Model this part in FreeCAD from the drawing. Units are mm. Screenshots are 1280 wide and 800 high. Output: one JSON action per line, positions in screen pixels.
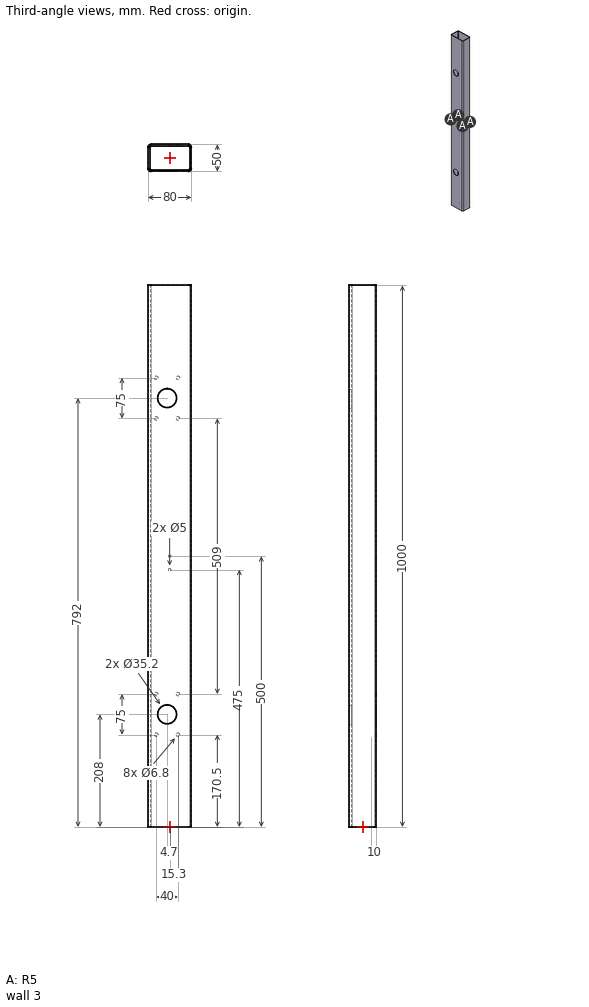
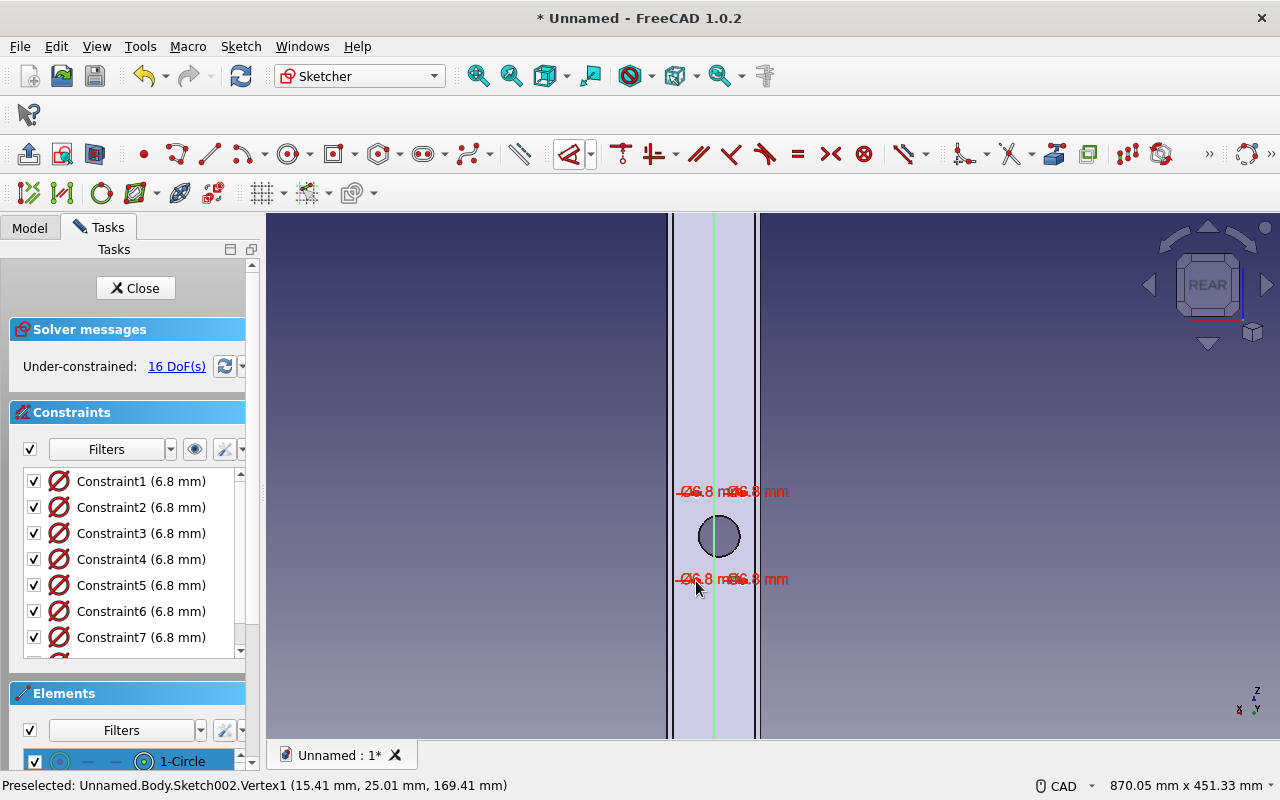
{"action": "left_click", "coordinate": [743, 581]}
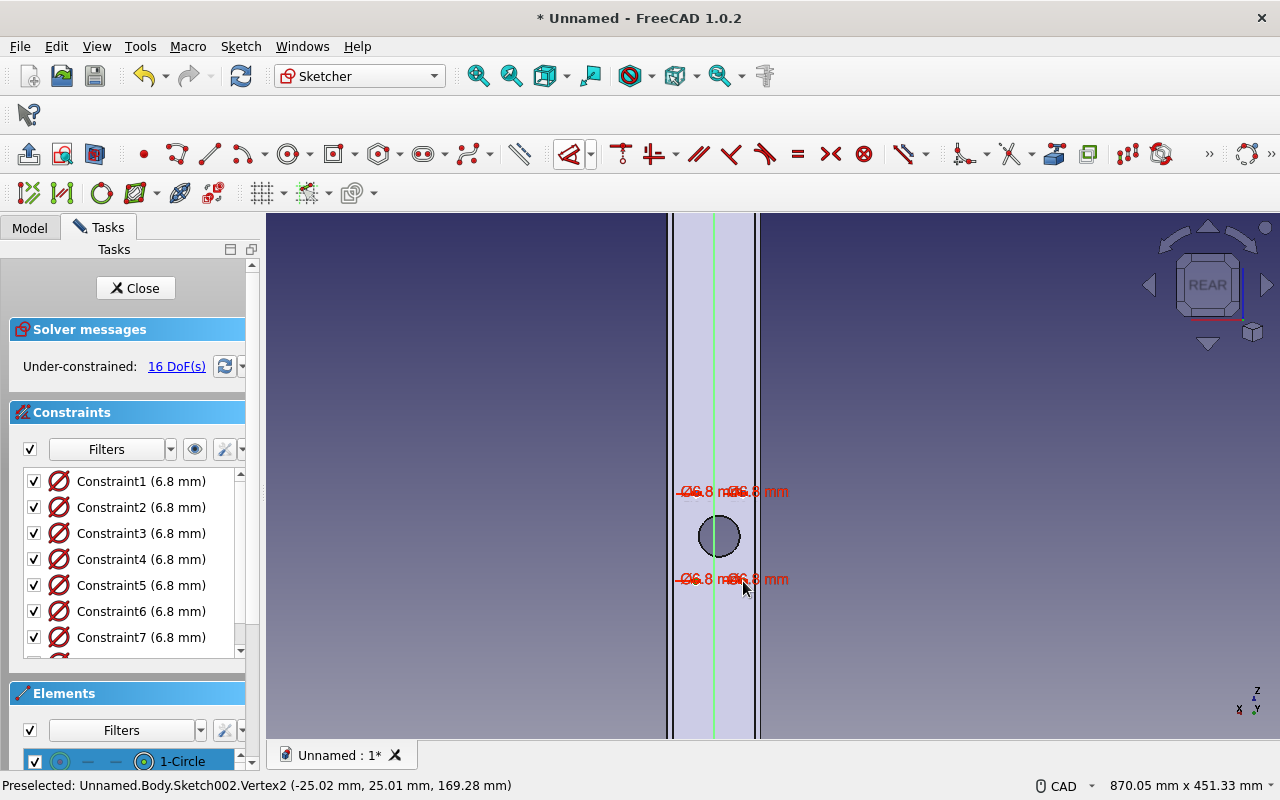
{"action": "left_click", "coordinate": [590, 154]}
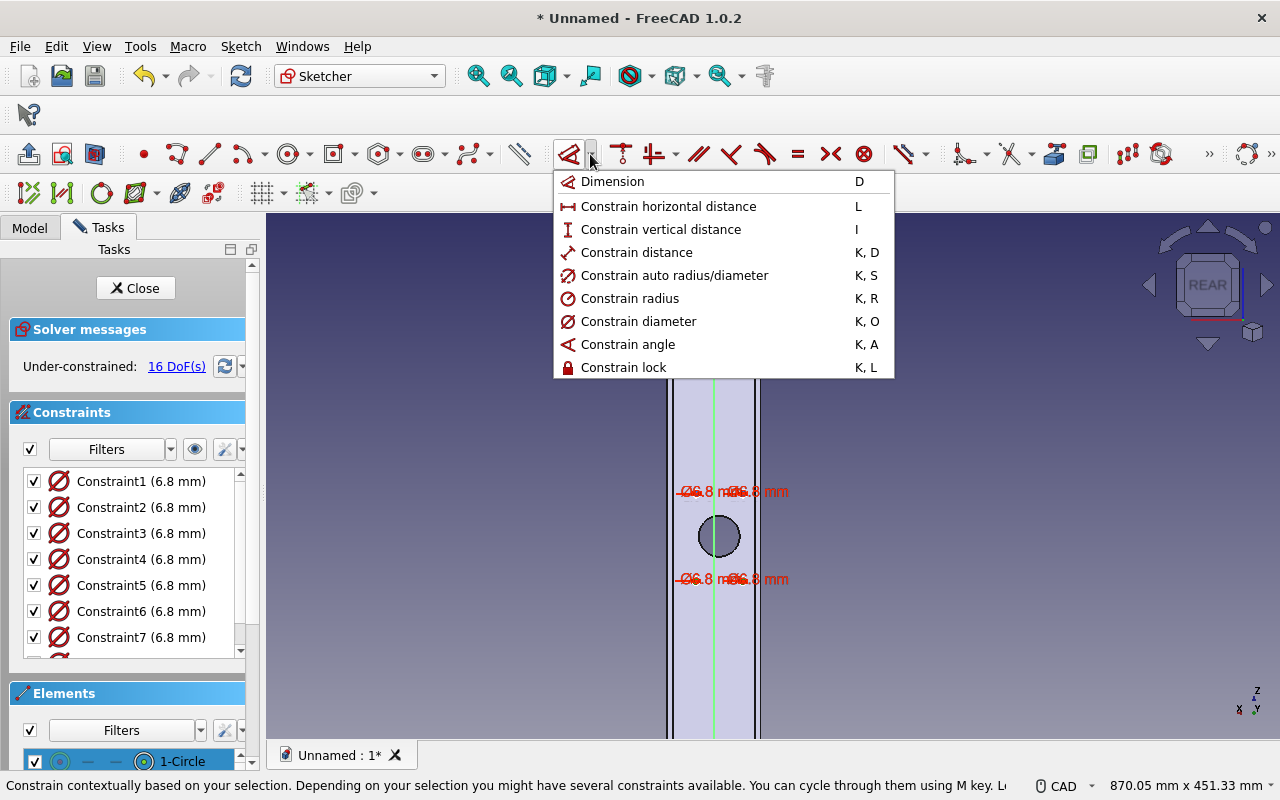
{"action": "left_click", "coordinate": [724, 206]}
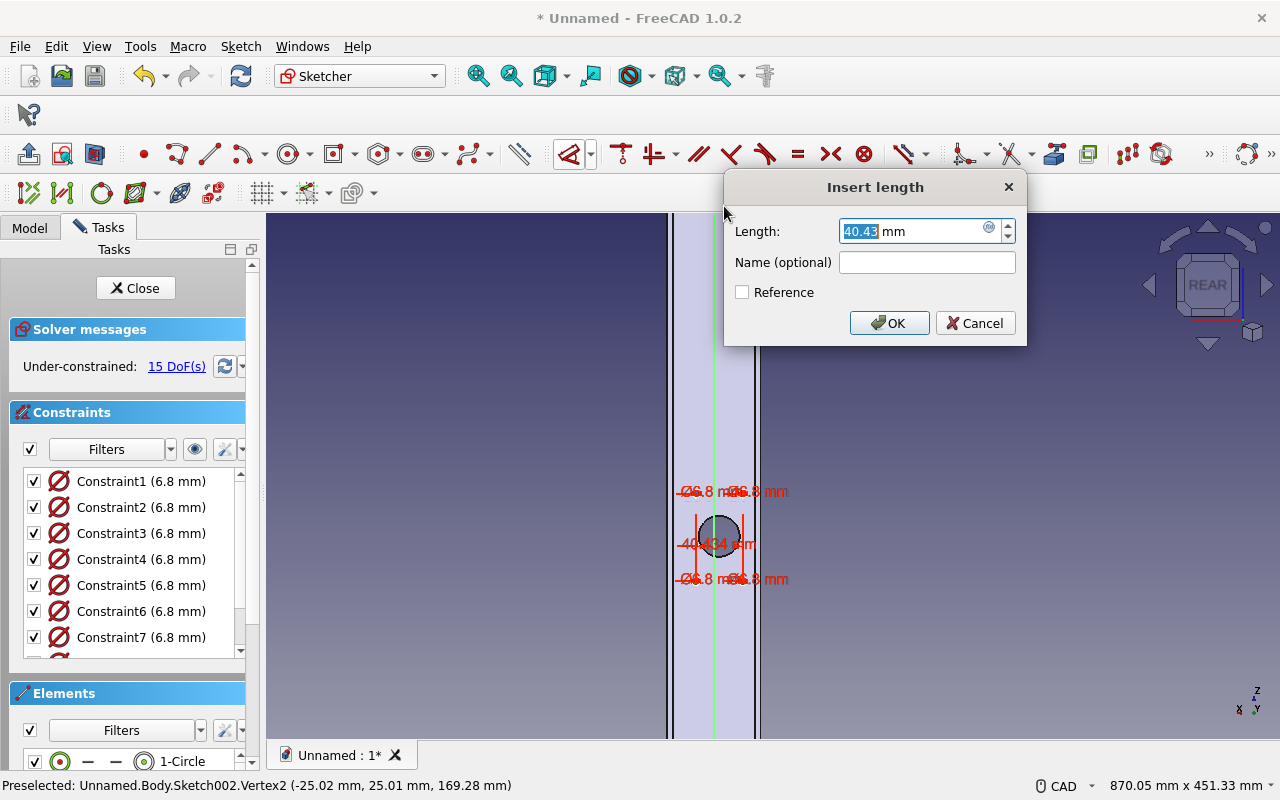
{"action": "type", "text": "40"}
{"action": "key", "text": "Return"}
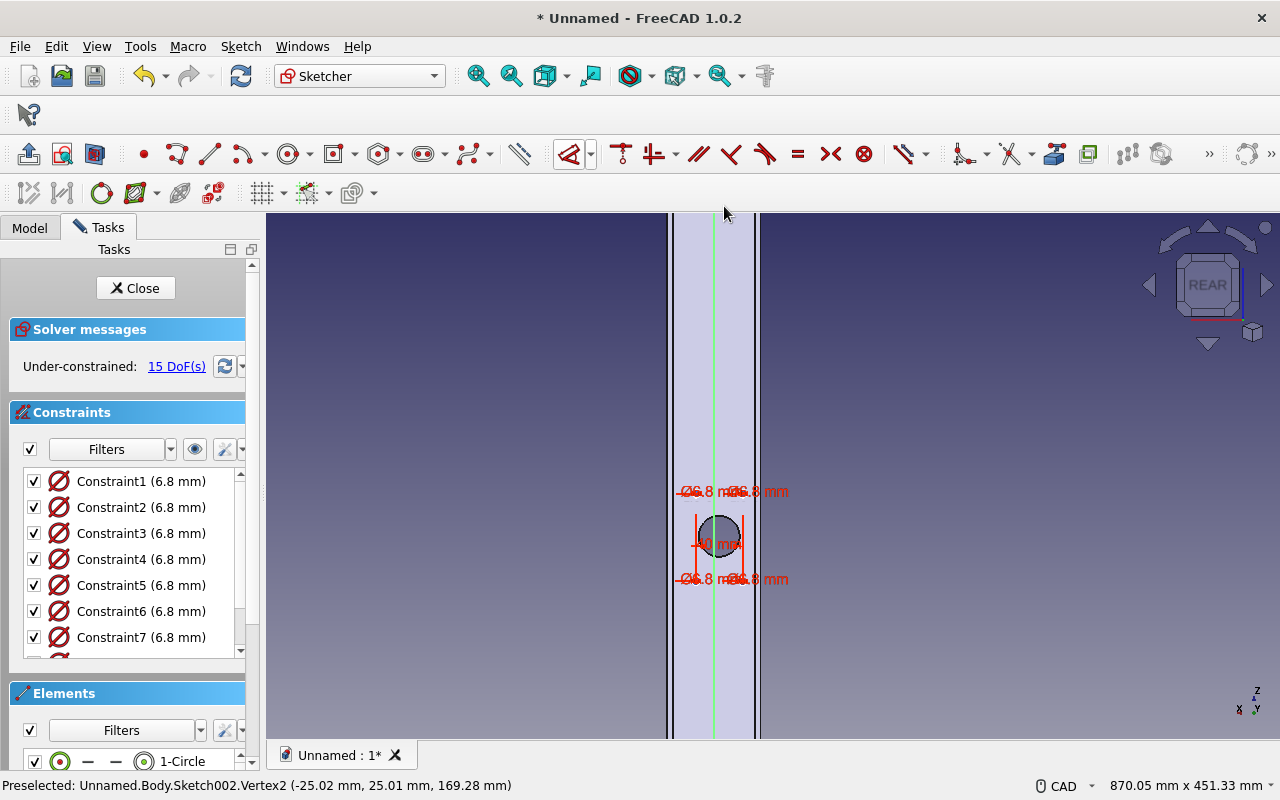
{"action": "left_click", "coordinate": [696, 581]}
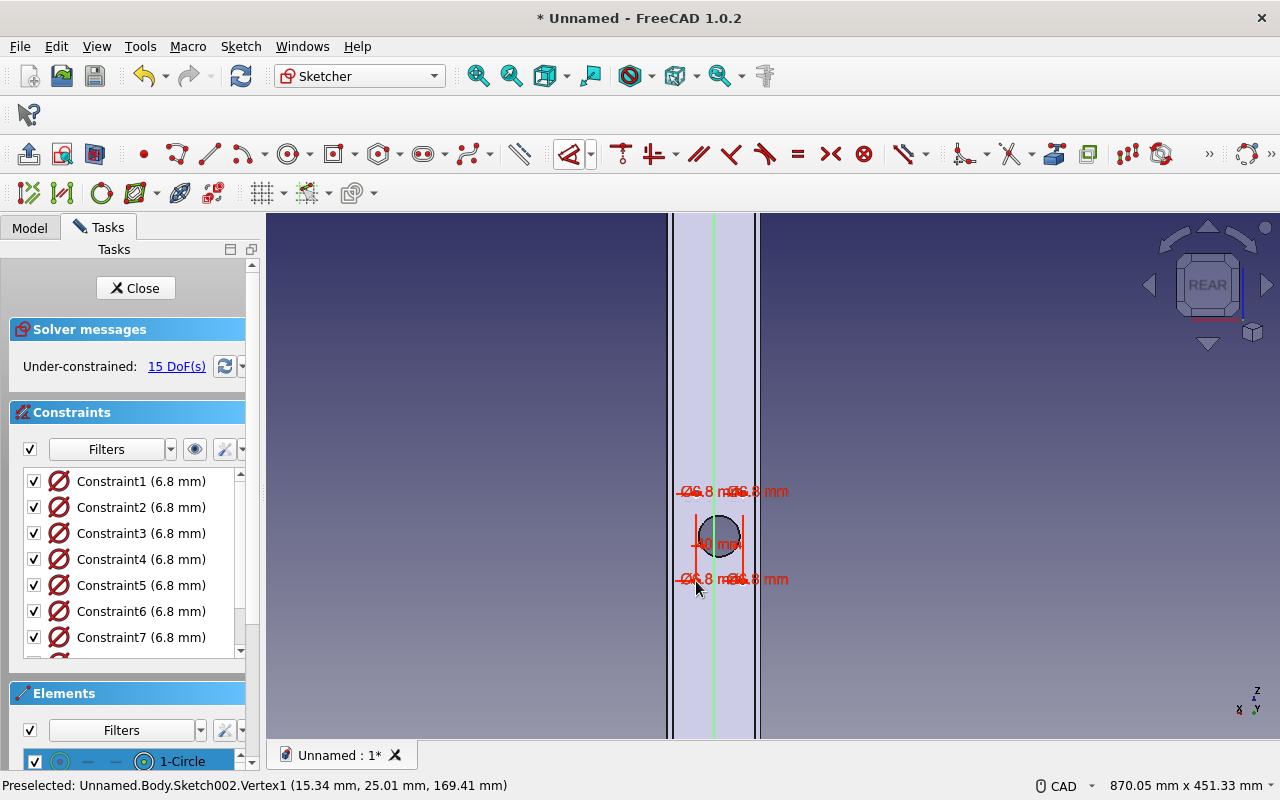
{"action": "left_click", "coordinate": [743, 494]}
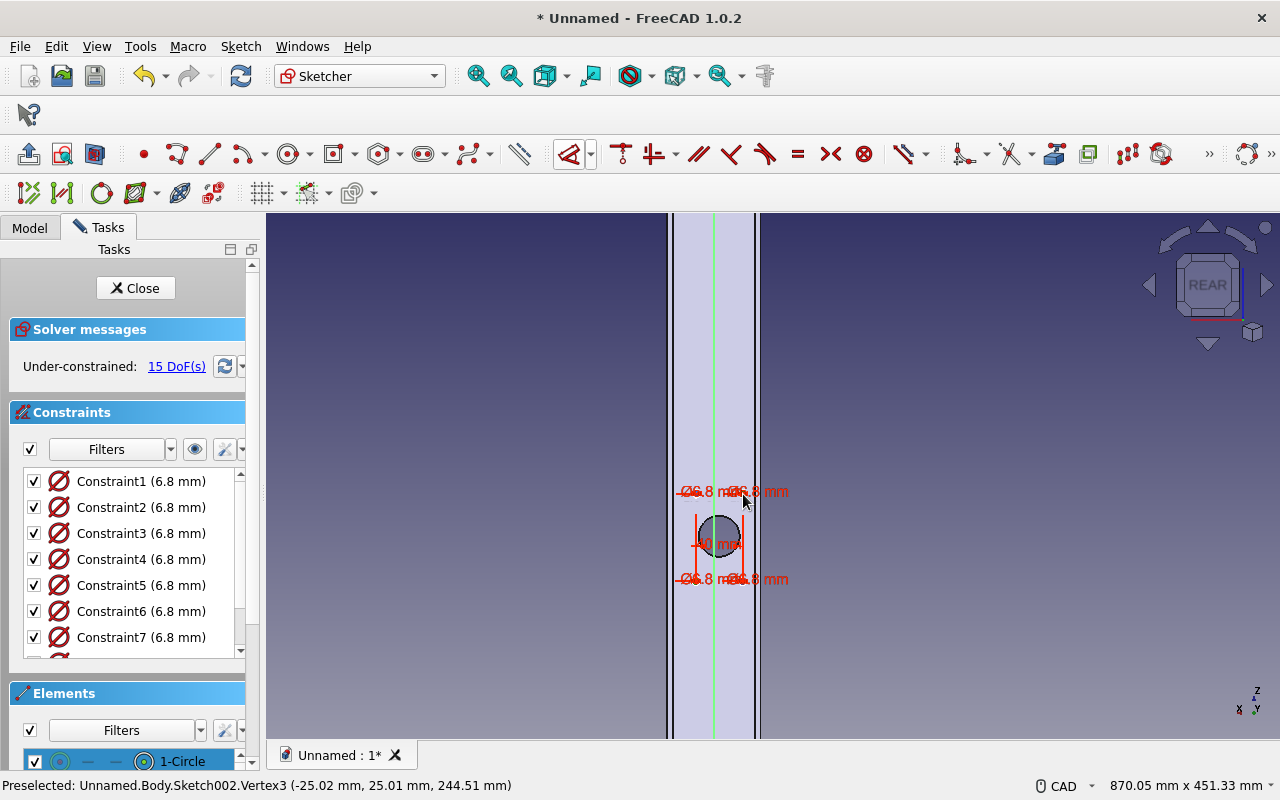
{"action": "left_click", "coordinate": [590, 154]}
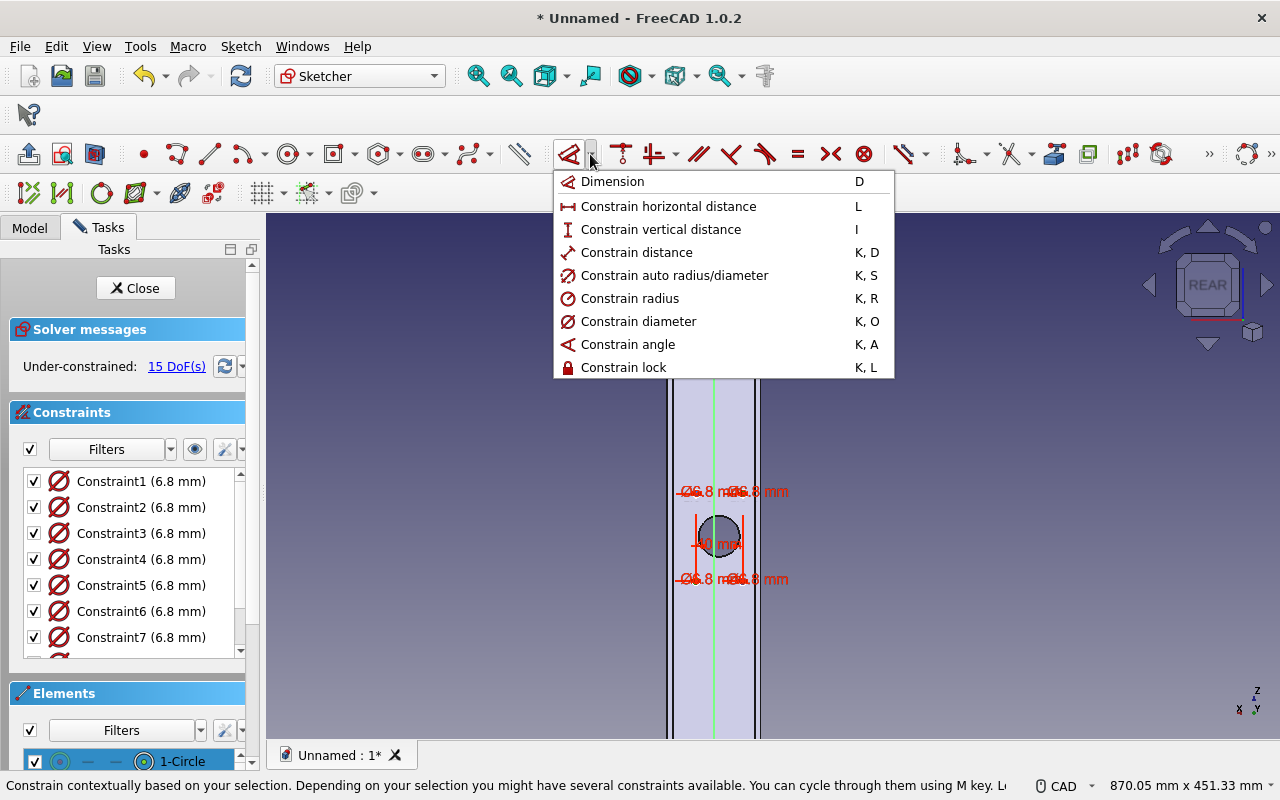
{"action": "left_click", "coordinate": [724, 206]}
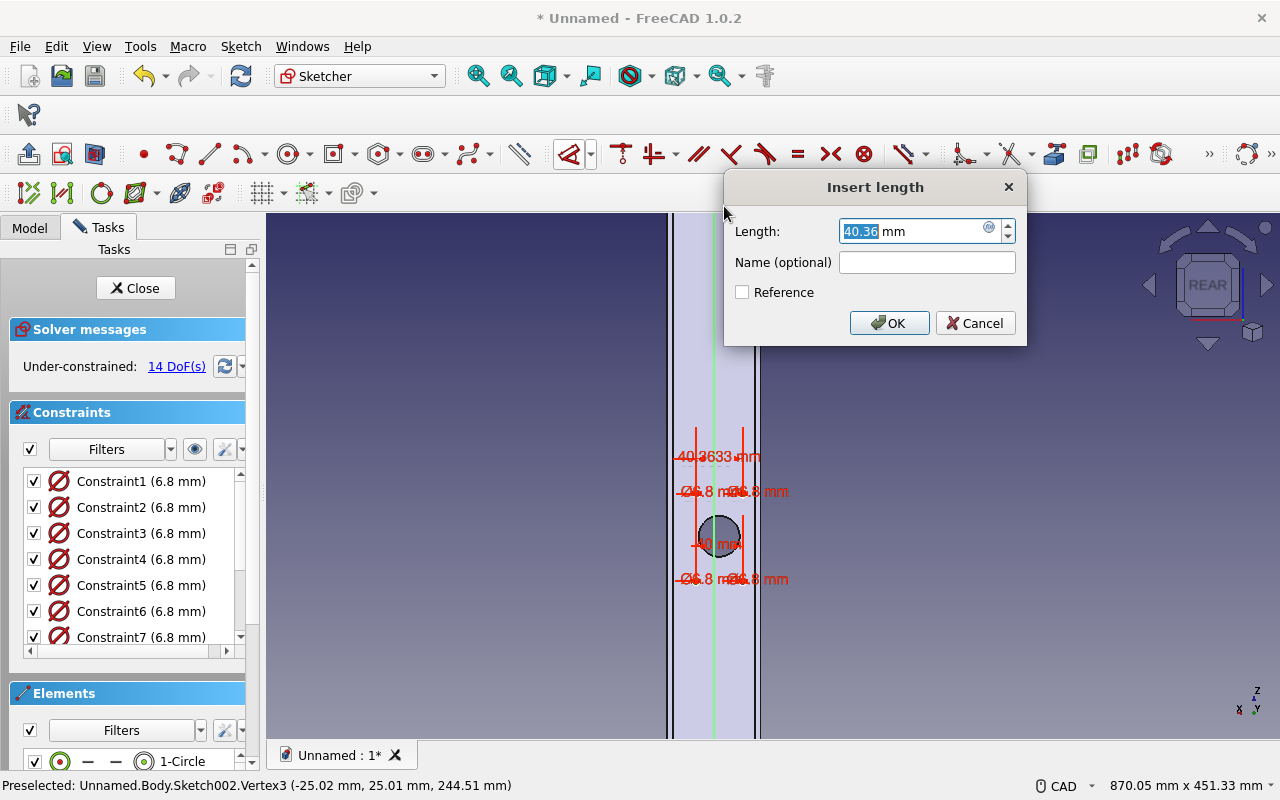
{"action": "type", "text": "40"}
{"action": "key", "text": "Return"}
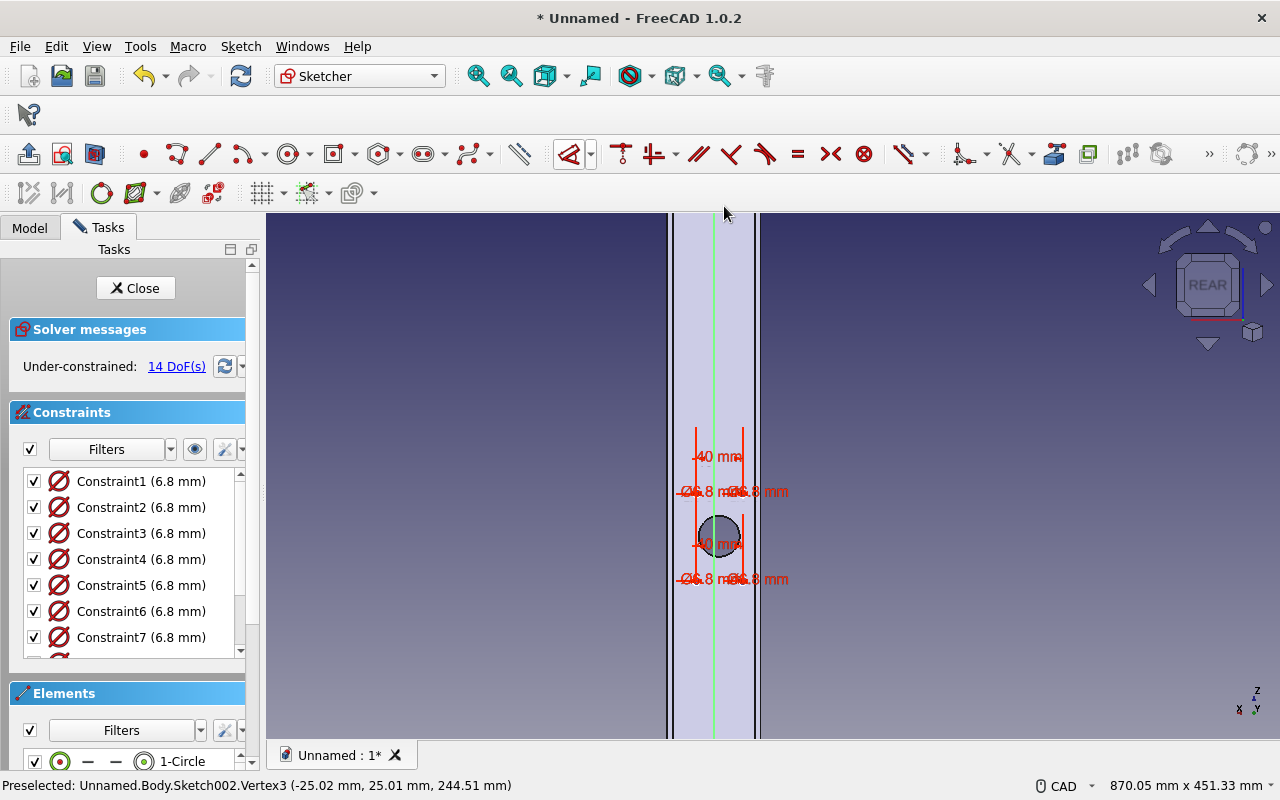
{"action": "left_click", "coordinate": [743, 581]}